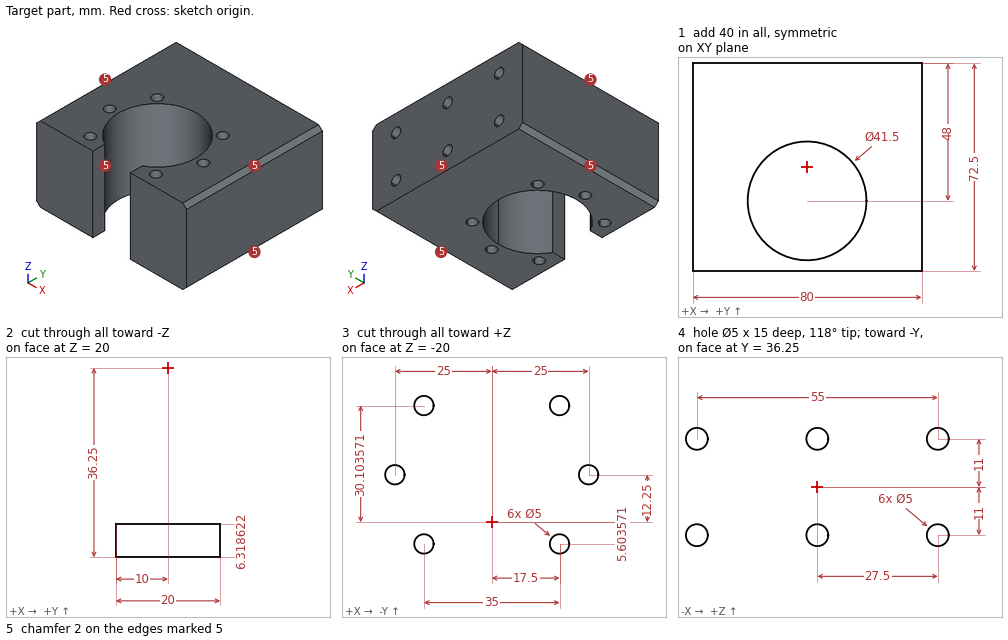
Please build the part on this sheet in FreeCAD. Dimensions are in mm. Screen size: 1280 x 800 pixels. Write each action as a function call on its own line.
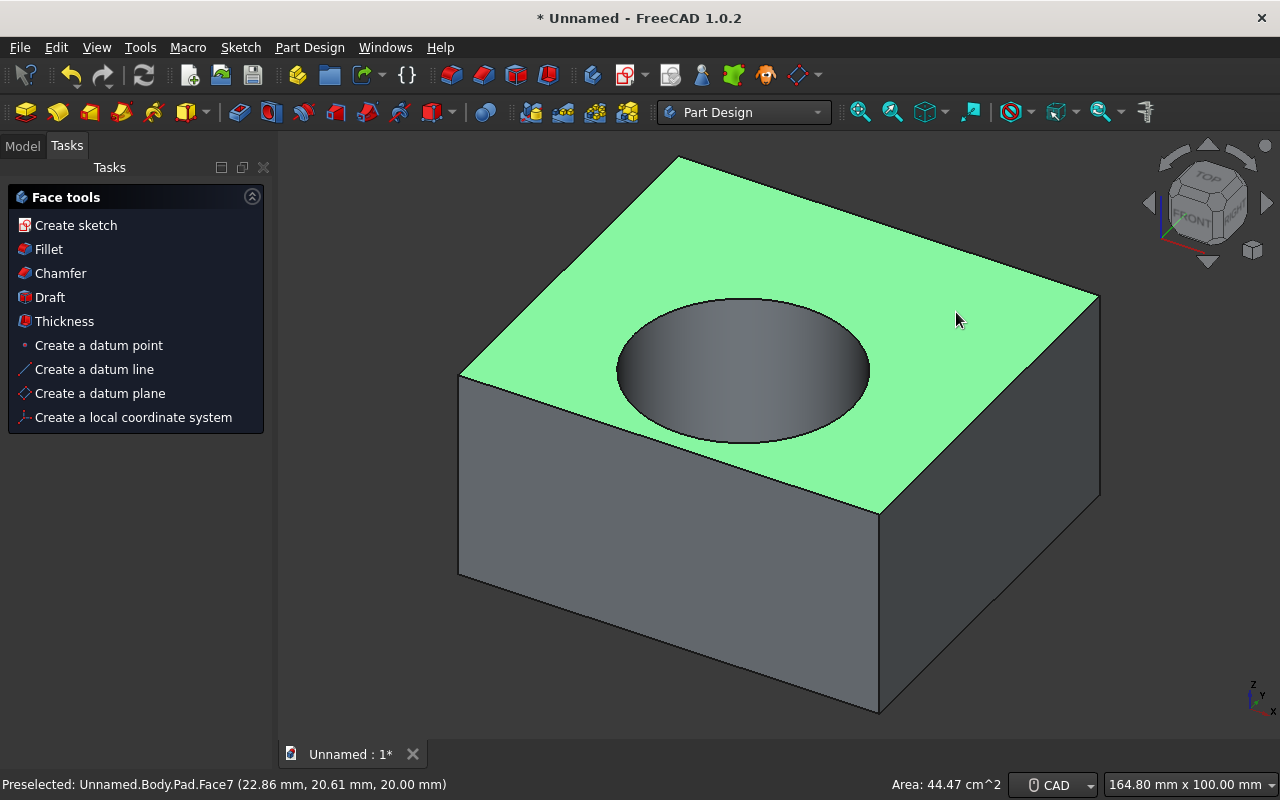
click(626, 76)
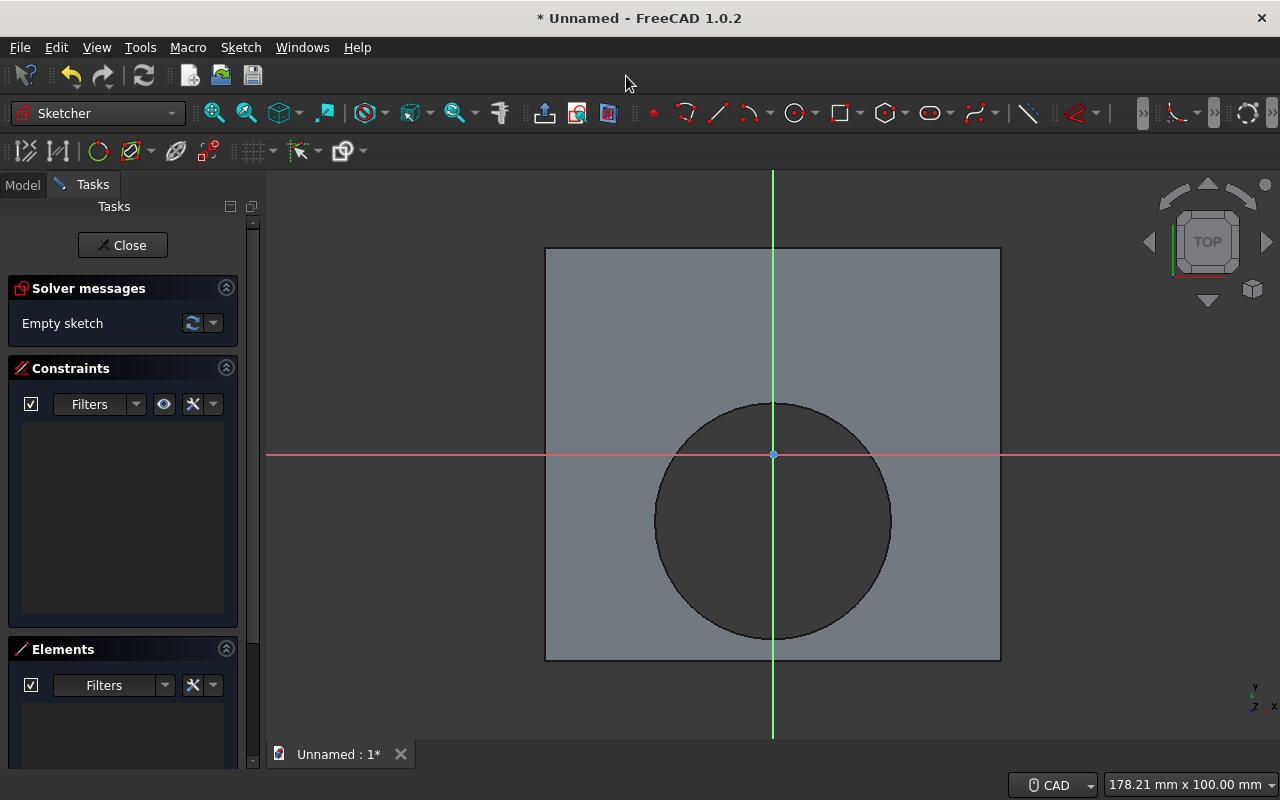
scroll(856, 683, up, 3)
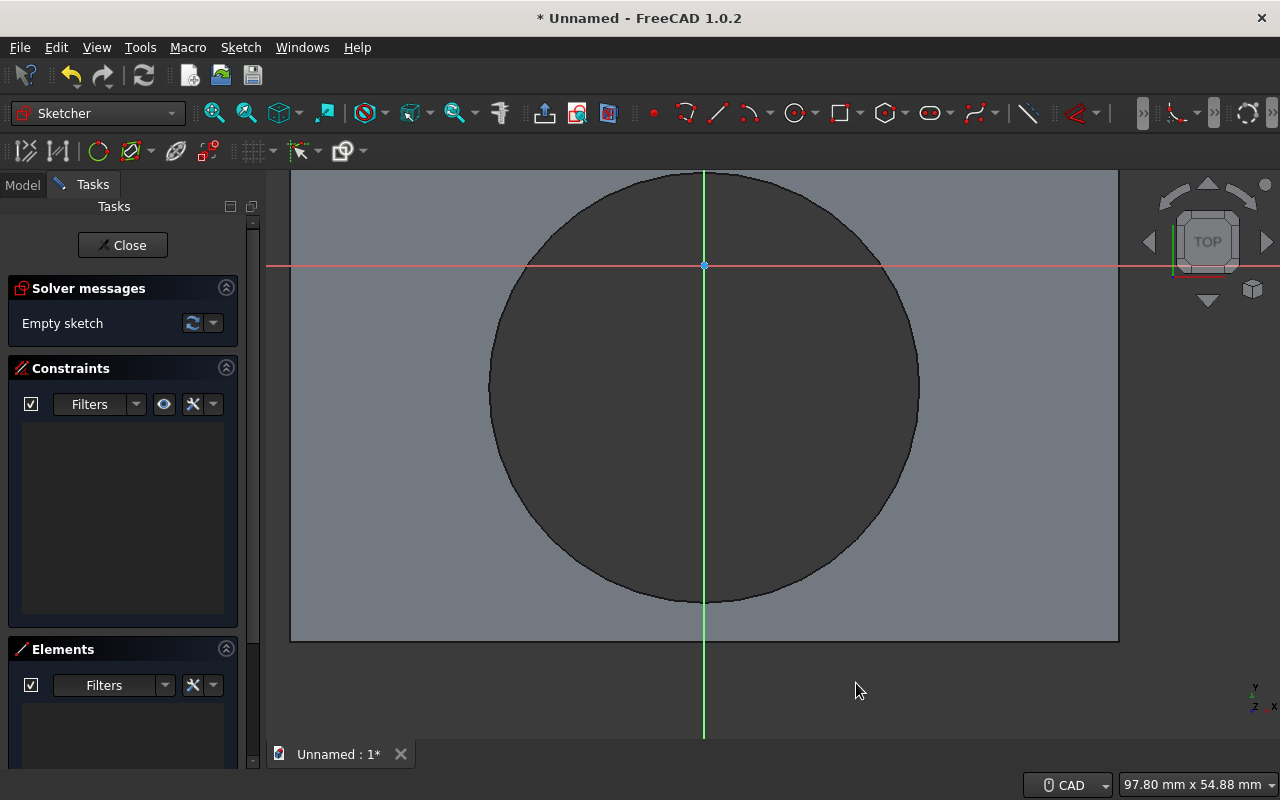
key(g)
key(r)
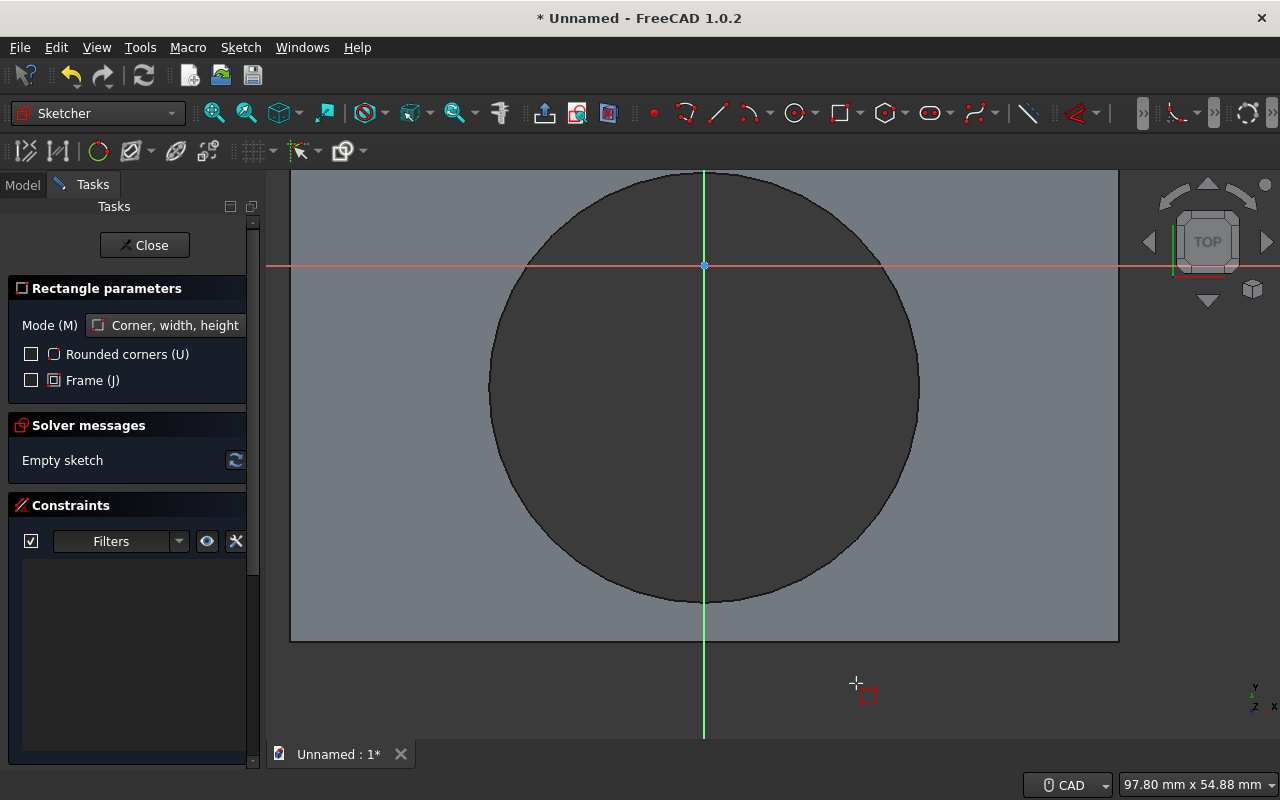
click(601, 576)
move(808, 642)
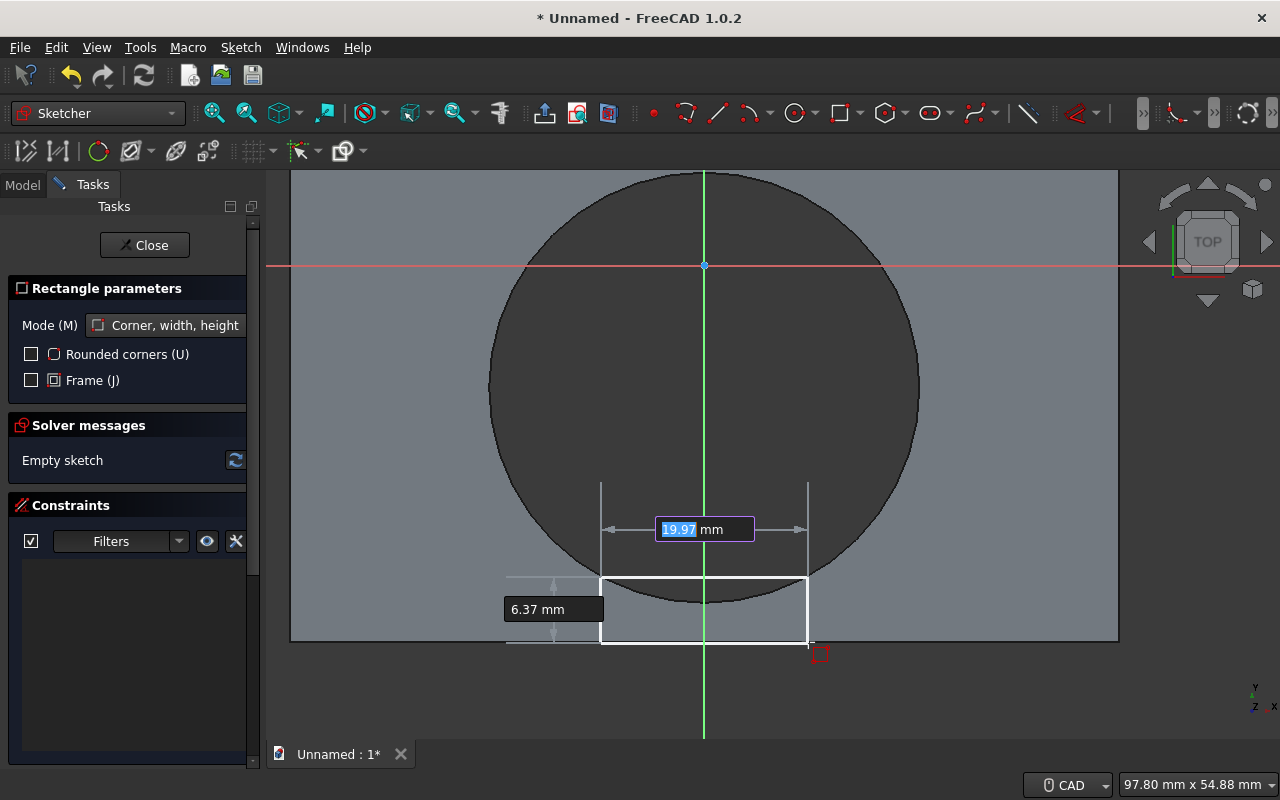
text(20)
key(Tab)
text(6.318622)
key(Return)
key(Escape)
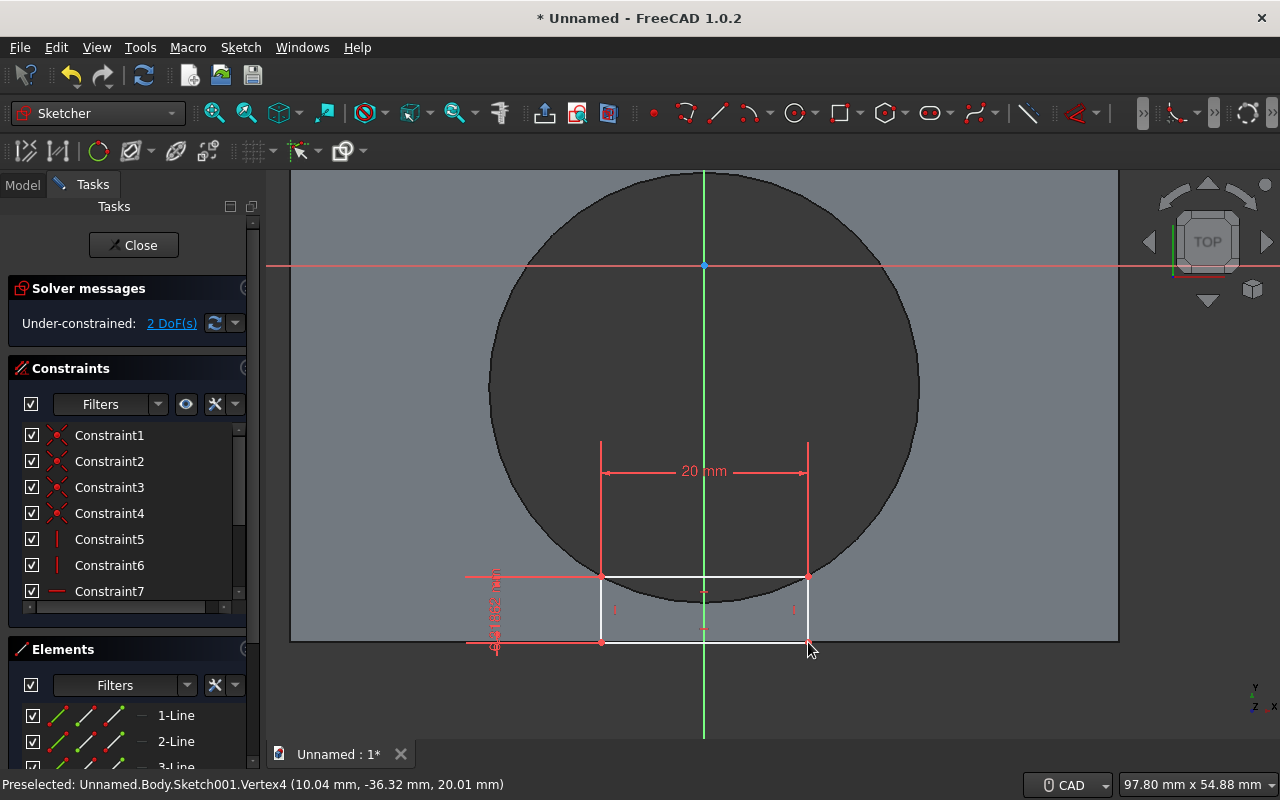
click(1076, 114)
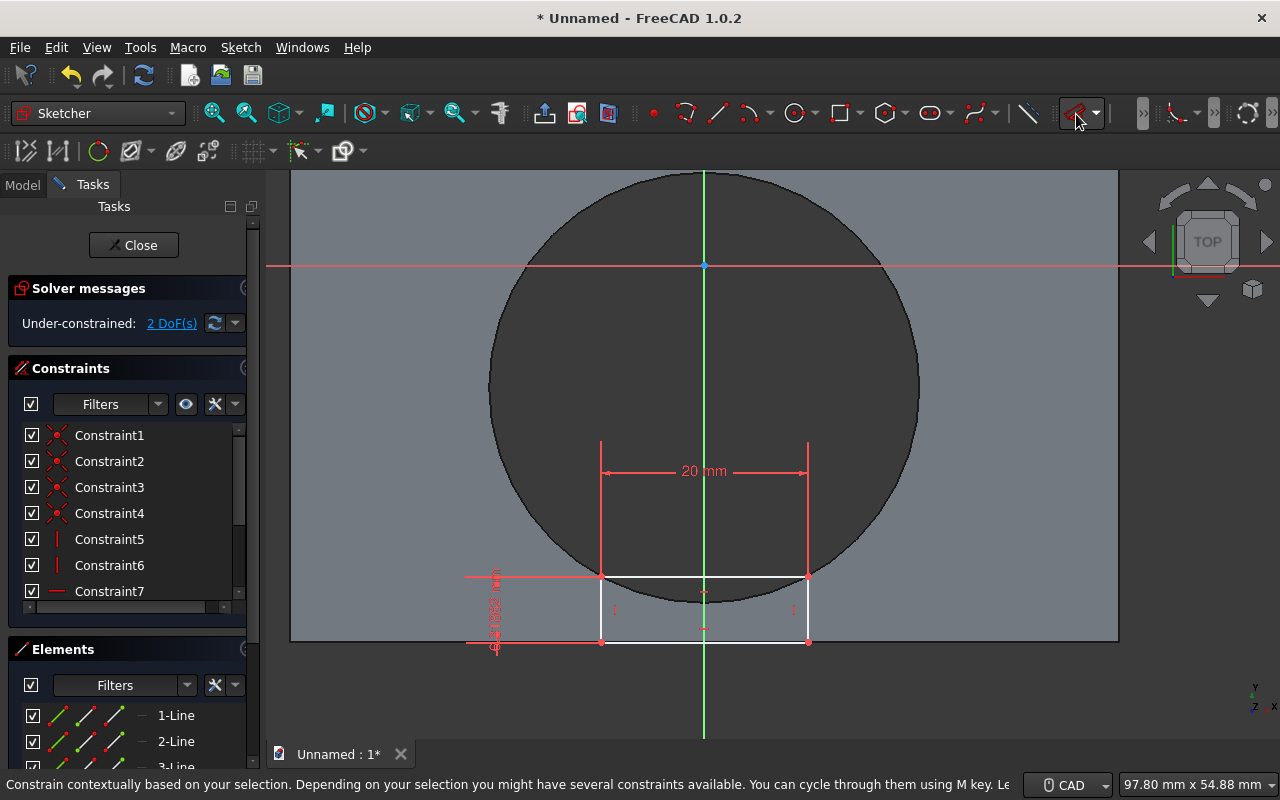
click(601, 577)
click(653, 232)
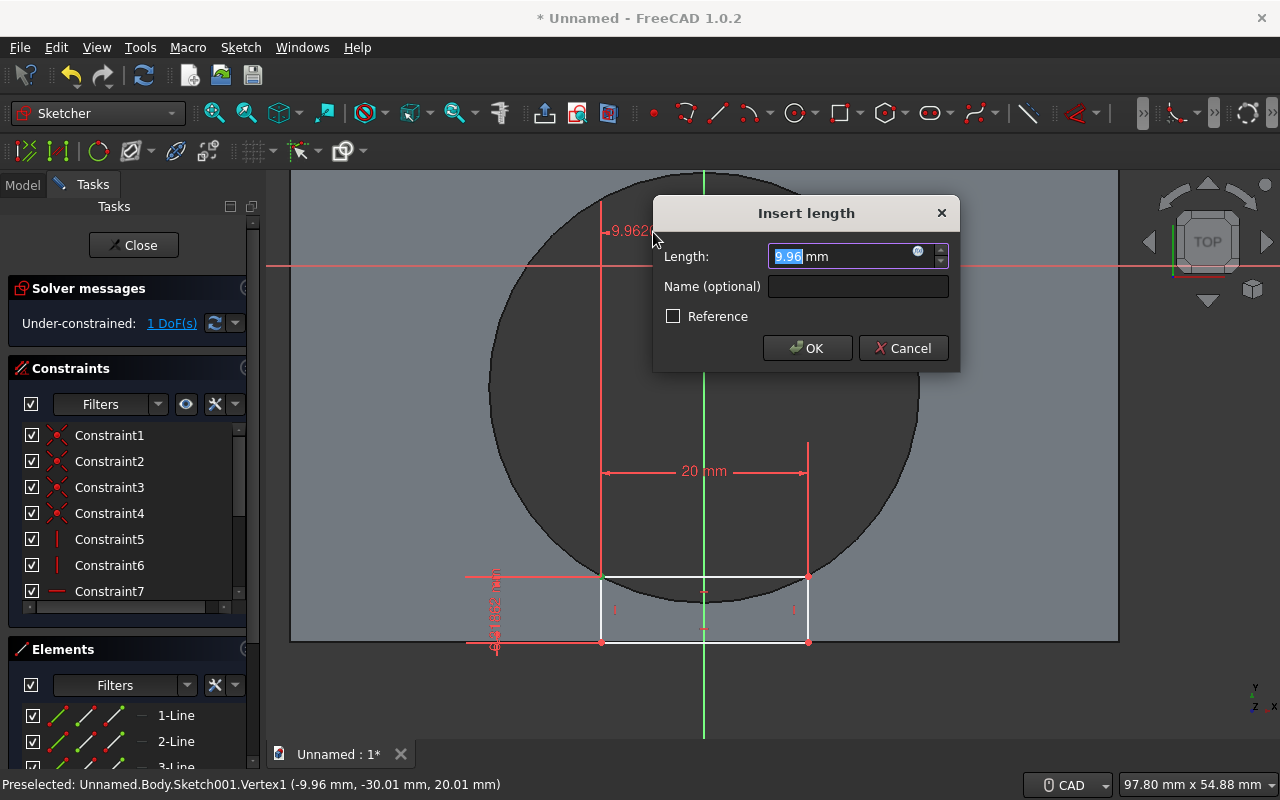
text(10)
key(Return)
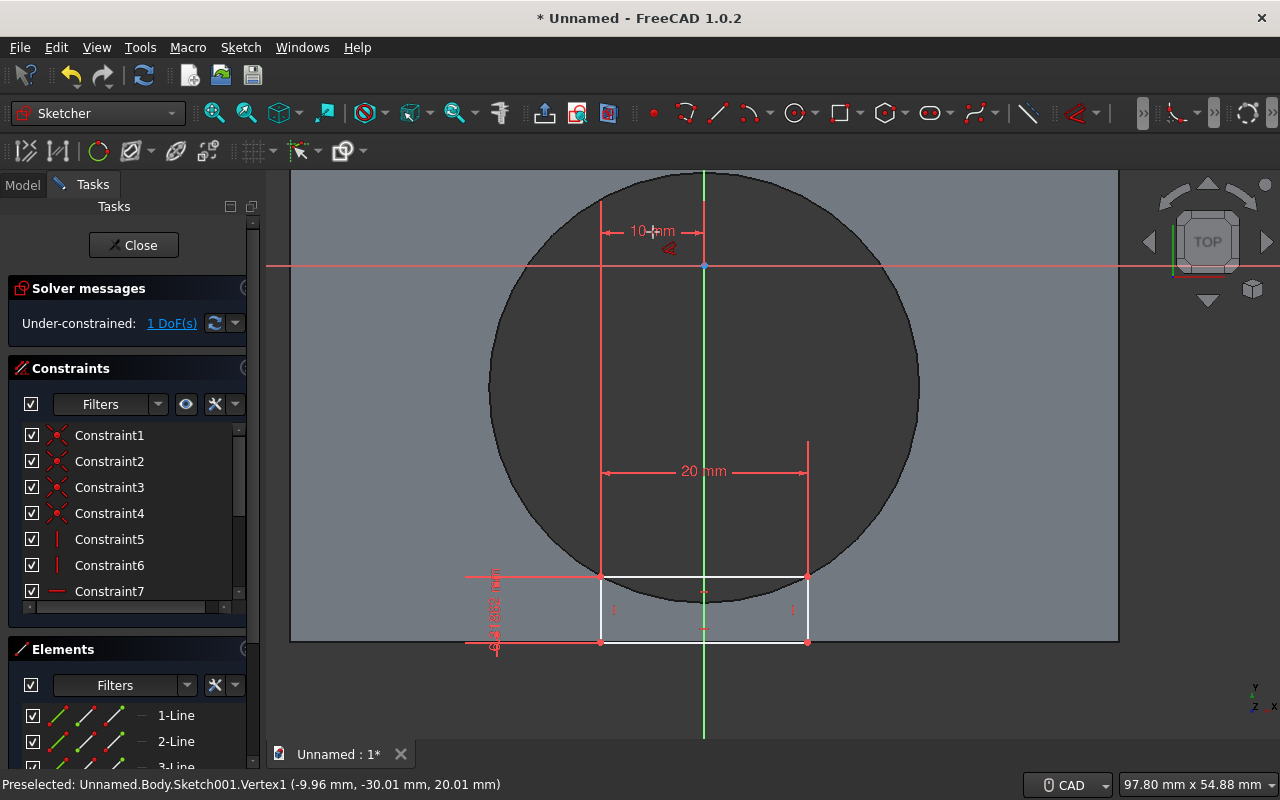
click(601, 643)
click(567, 454)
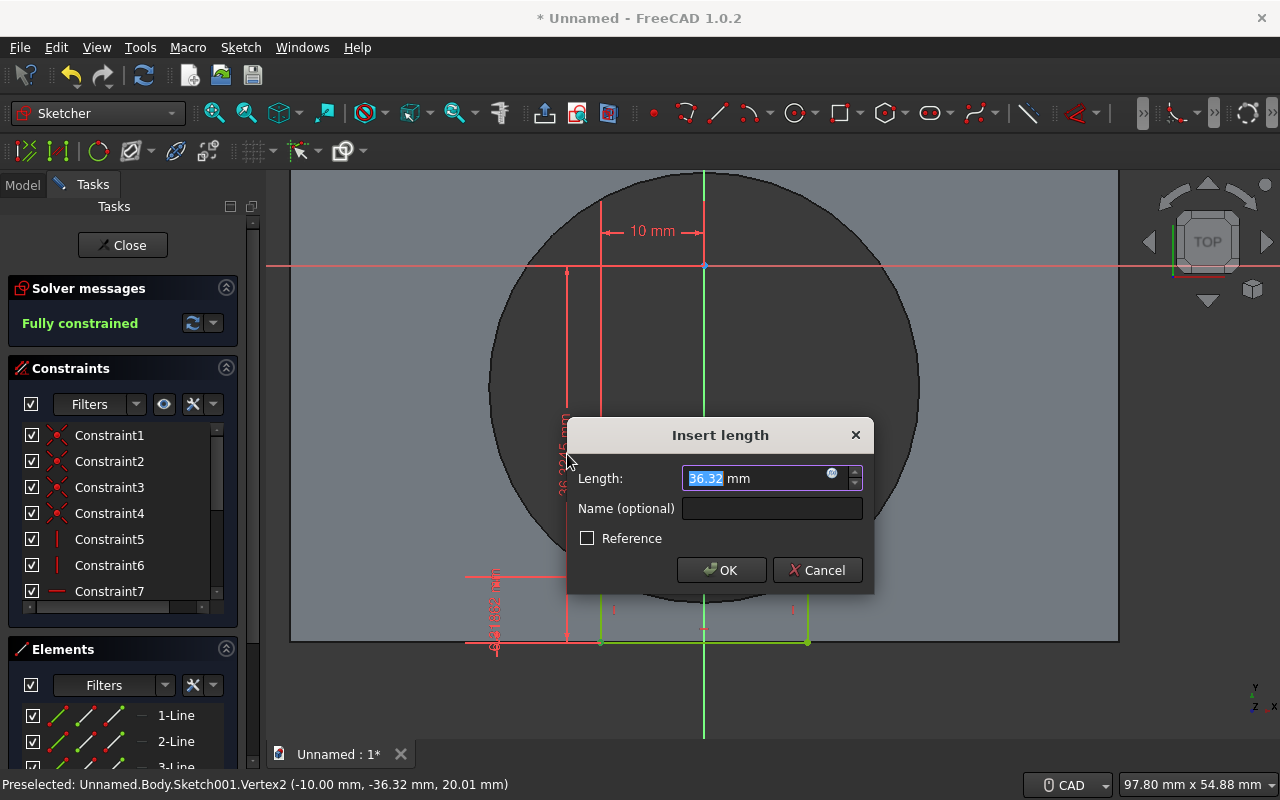
text(36.25)
key(Return)
key(Escape)